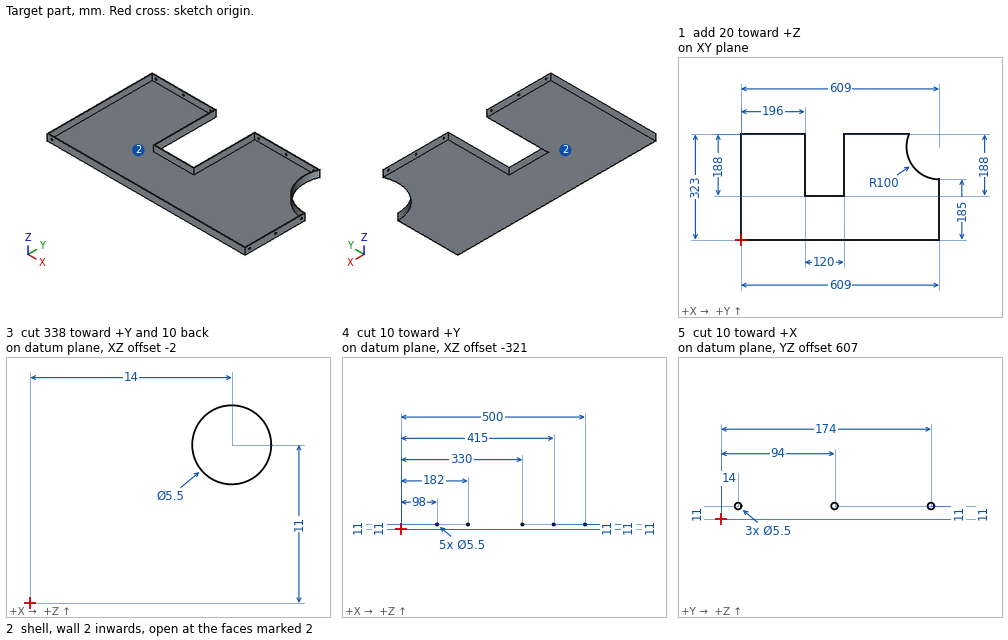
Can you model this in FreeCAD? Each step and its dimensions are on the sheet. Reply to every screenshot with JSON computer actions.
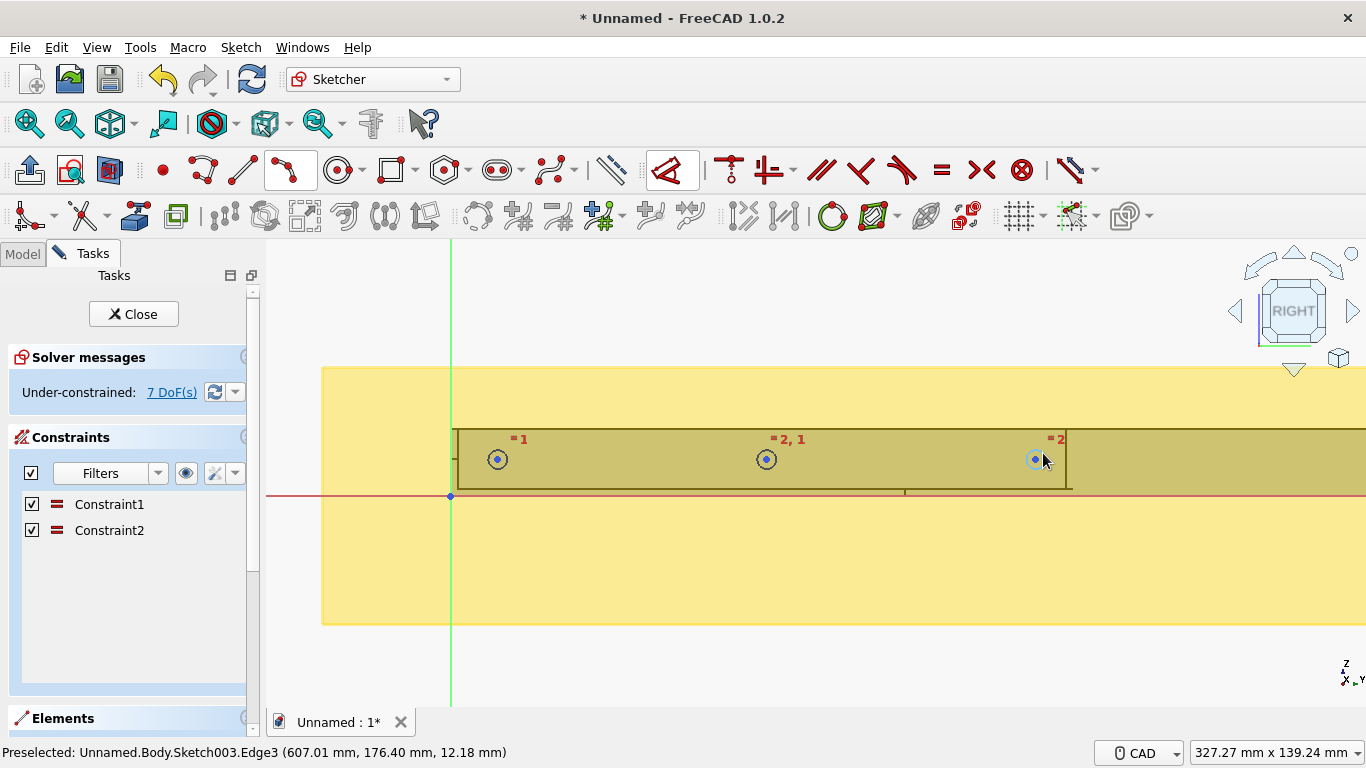
{"action": "scroll", "coordinate": [504, 453], "scroll_direction": "up", "scroll_amount": 4}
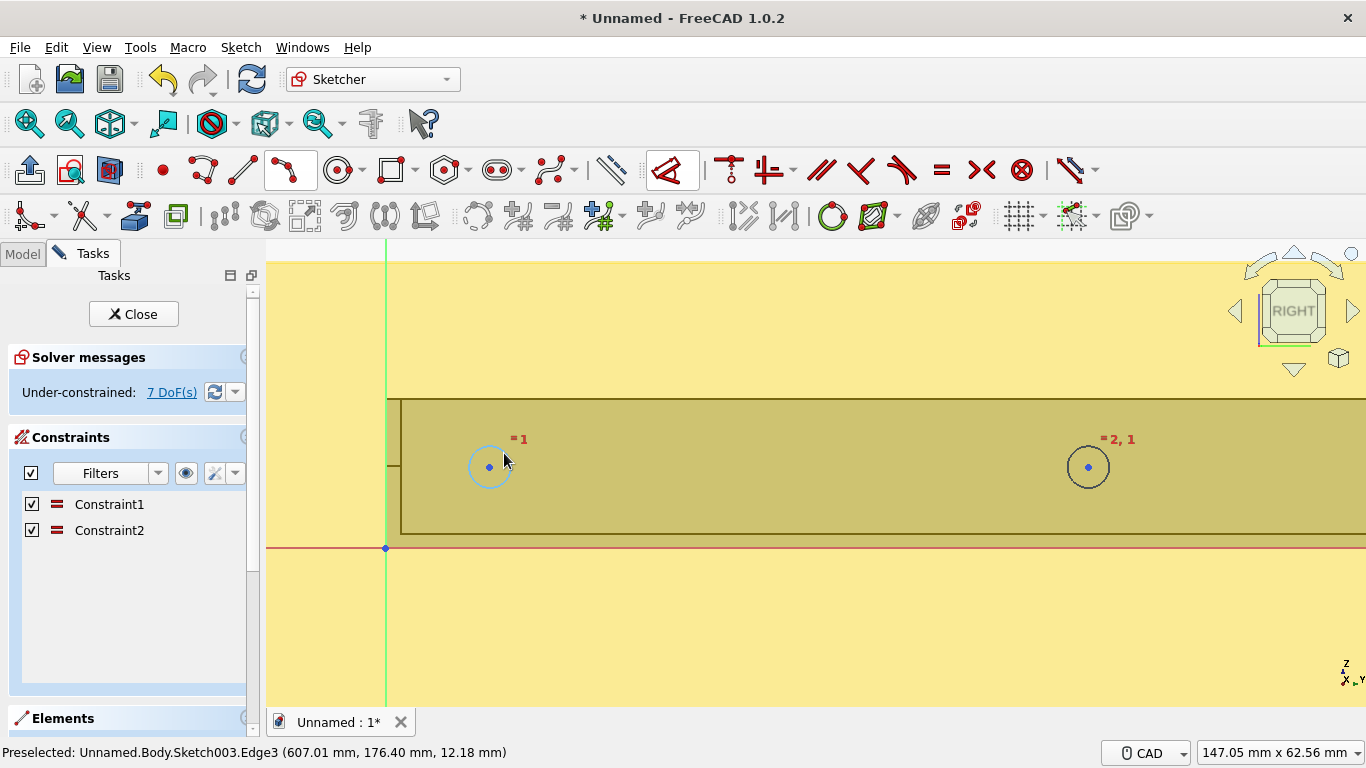
{"action": "left_click", "coordinate": [505, 452]}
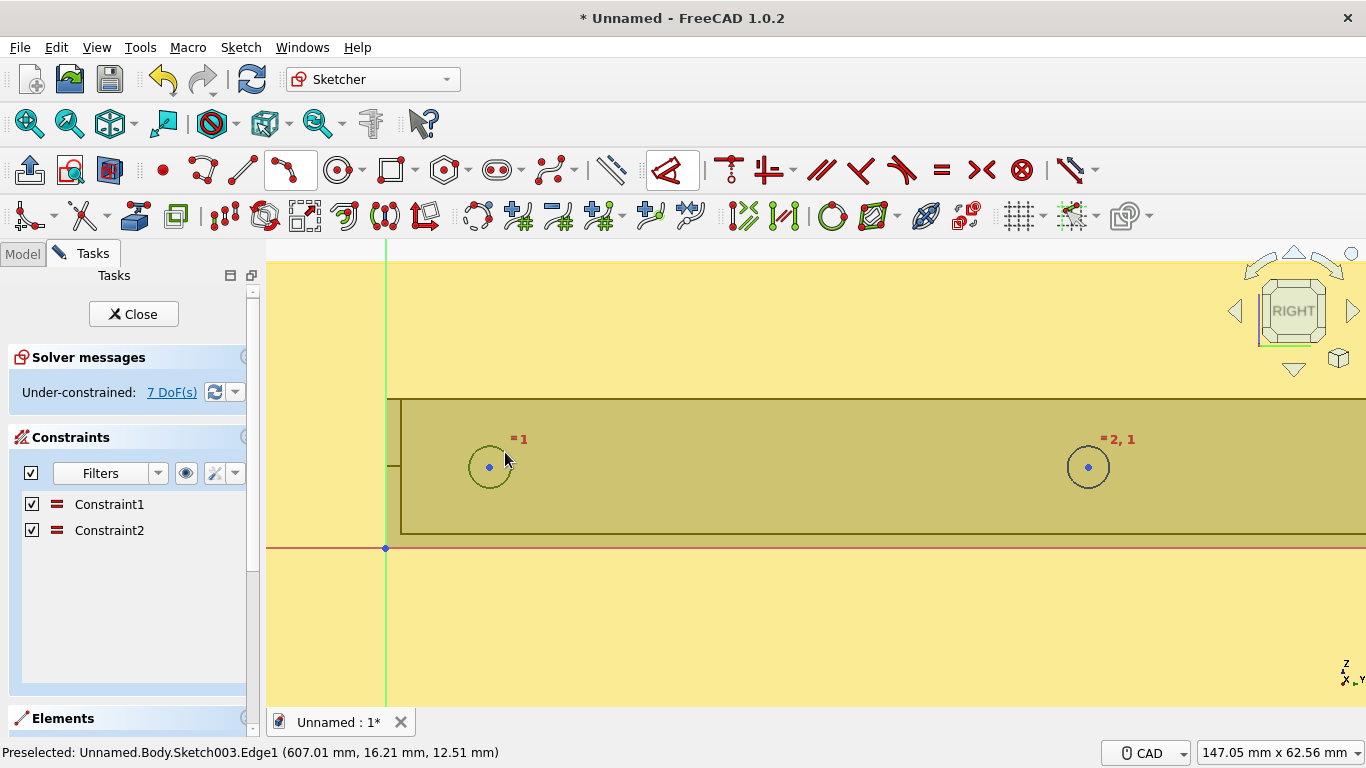
{"action": "key", "text": "k o"}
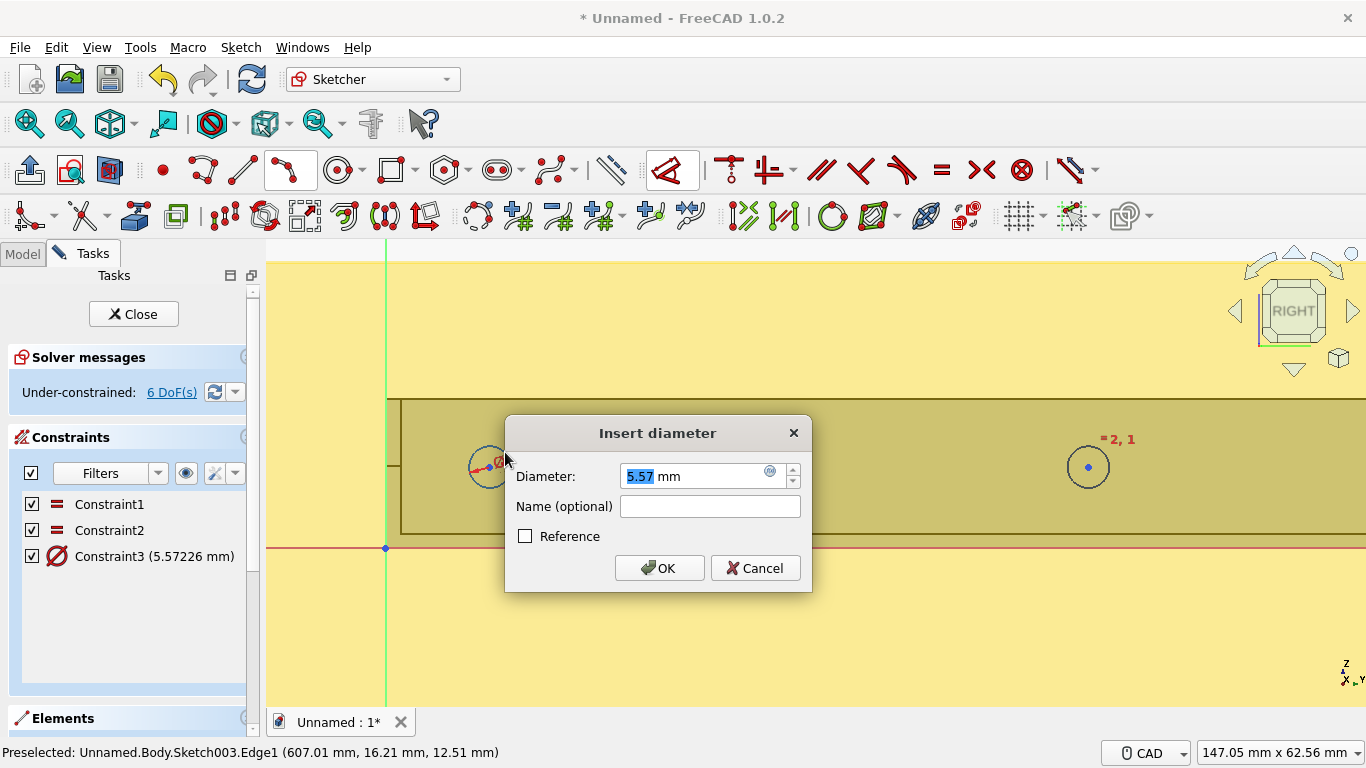
{"action": "type", "text": "5.5"}
{"action": "key", "text": "Return"}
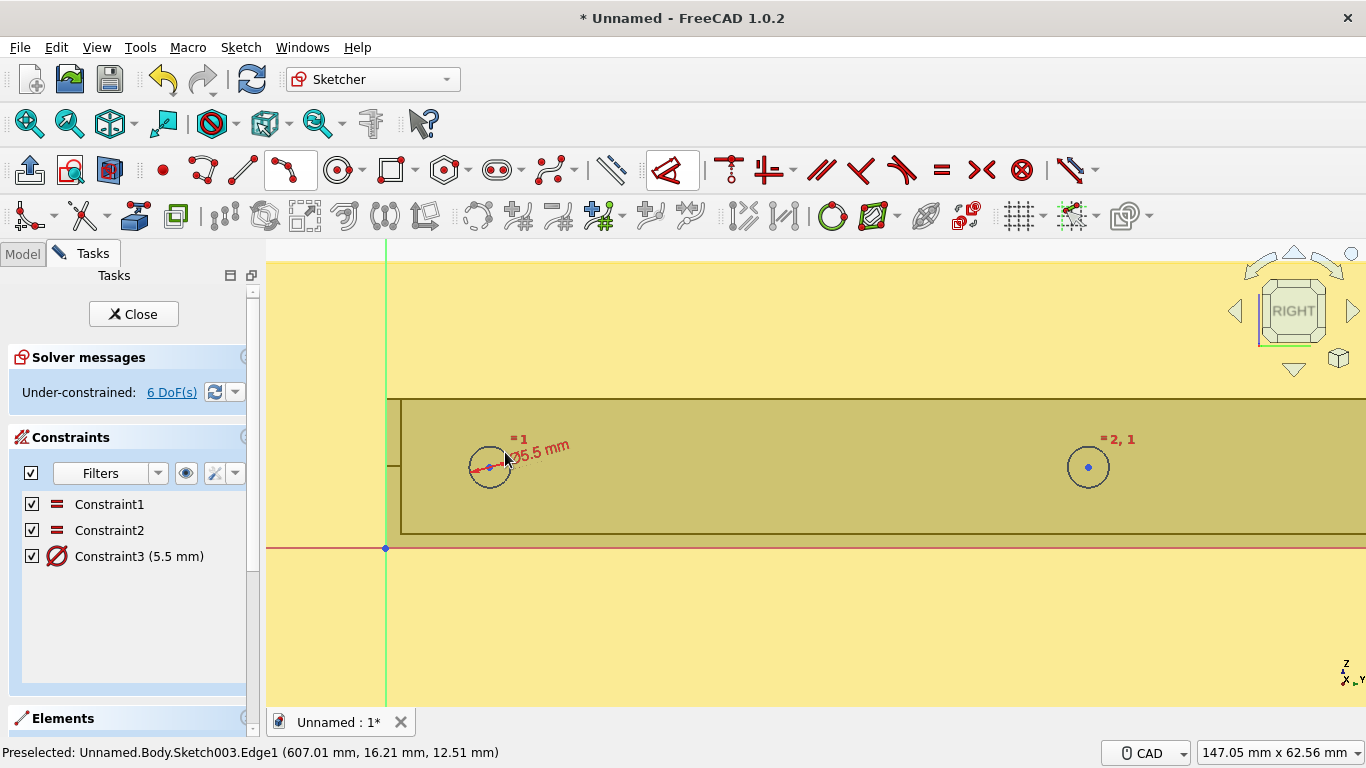
{"action": "left_click", "coordinate": [490, 467]}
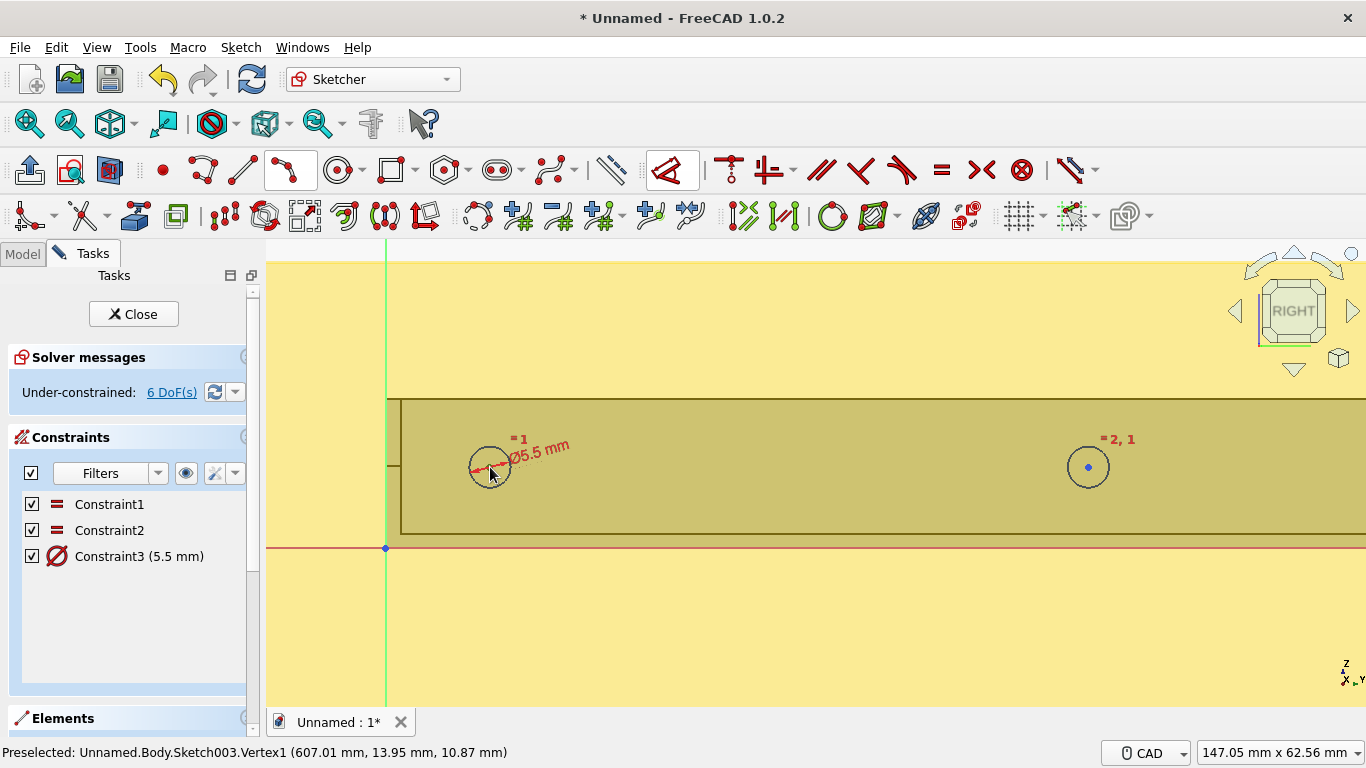
{"action": "key", "text": "l"}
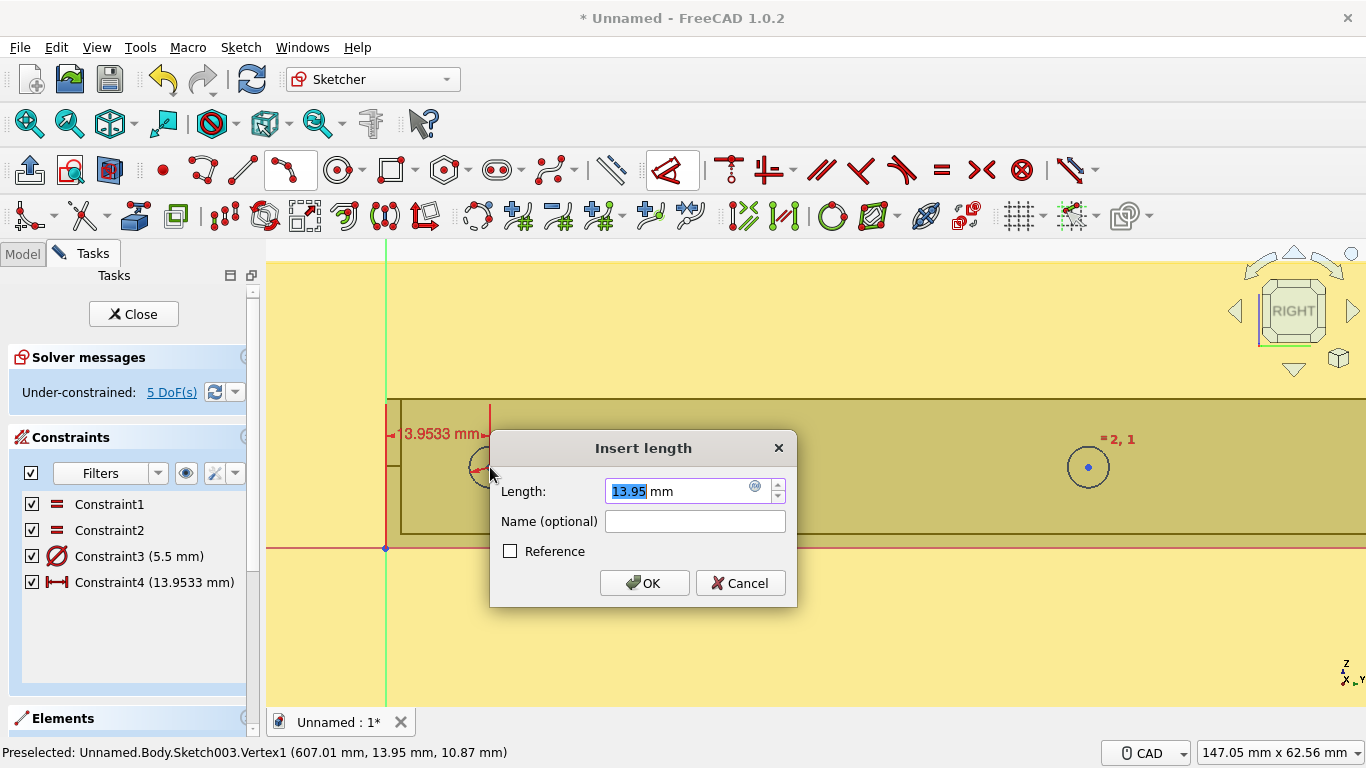
{"action": "type", "text": "14"}
{"action": "key", "text": "Return"}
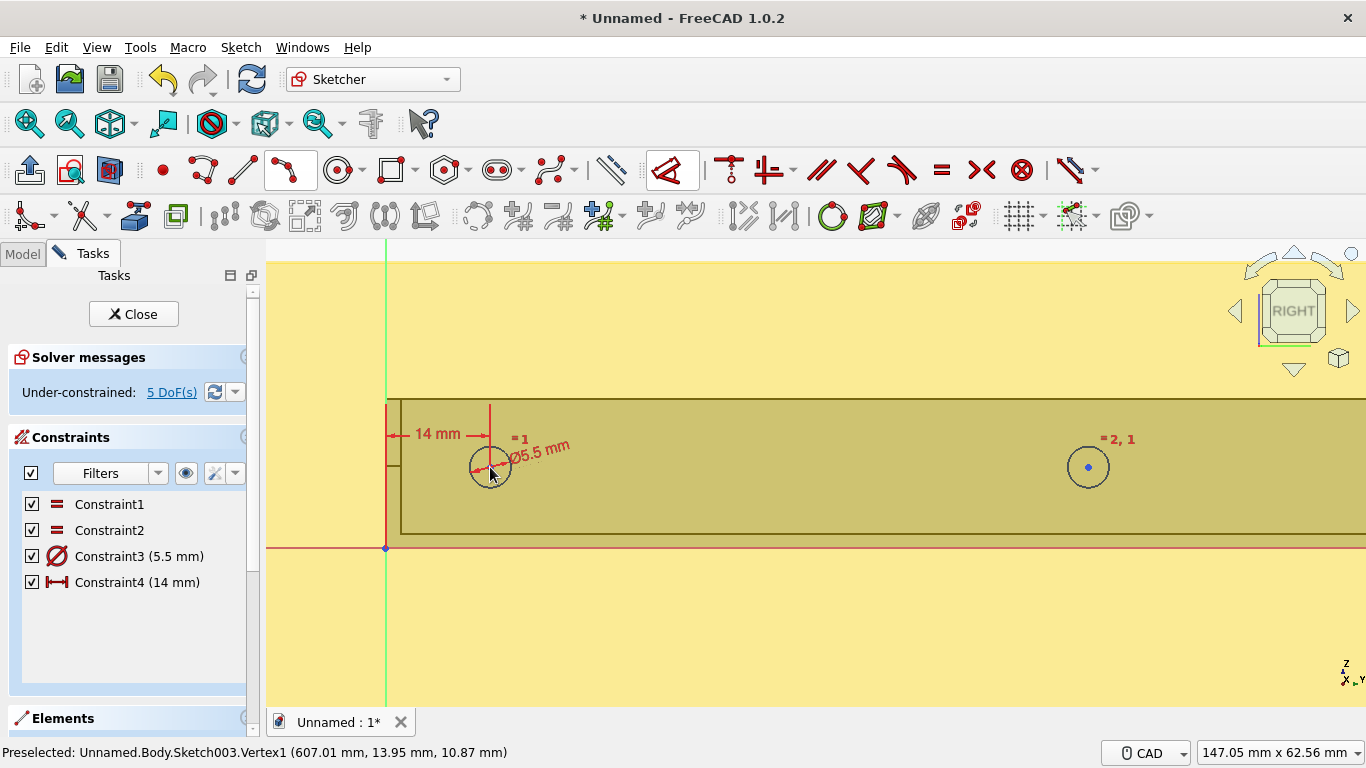
{"action": "left_click", "coordinate": [490, 467]}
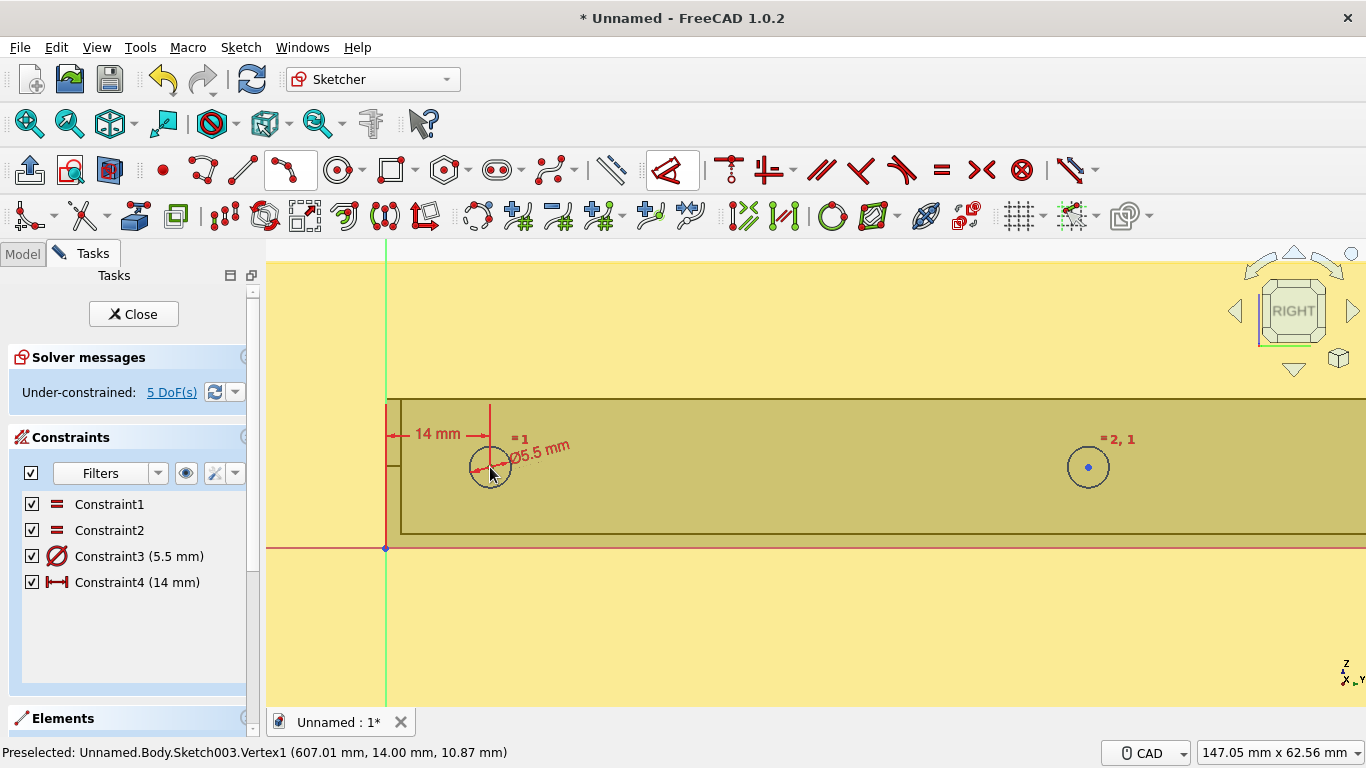
{"action": "key", "text": "i"}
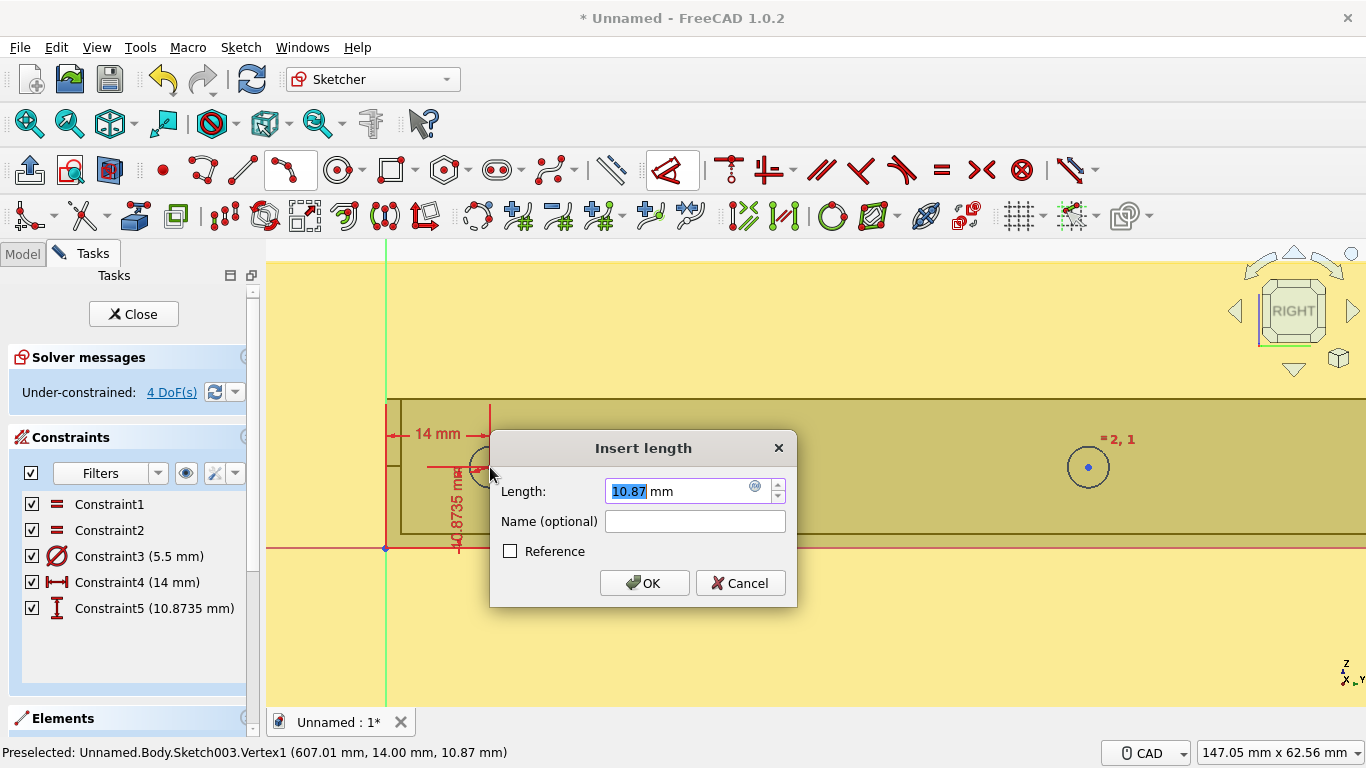
{"action": "type", "text": "11"}
{"action": "key", "text": "Return"}